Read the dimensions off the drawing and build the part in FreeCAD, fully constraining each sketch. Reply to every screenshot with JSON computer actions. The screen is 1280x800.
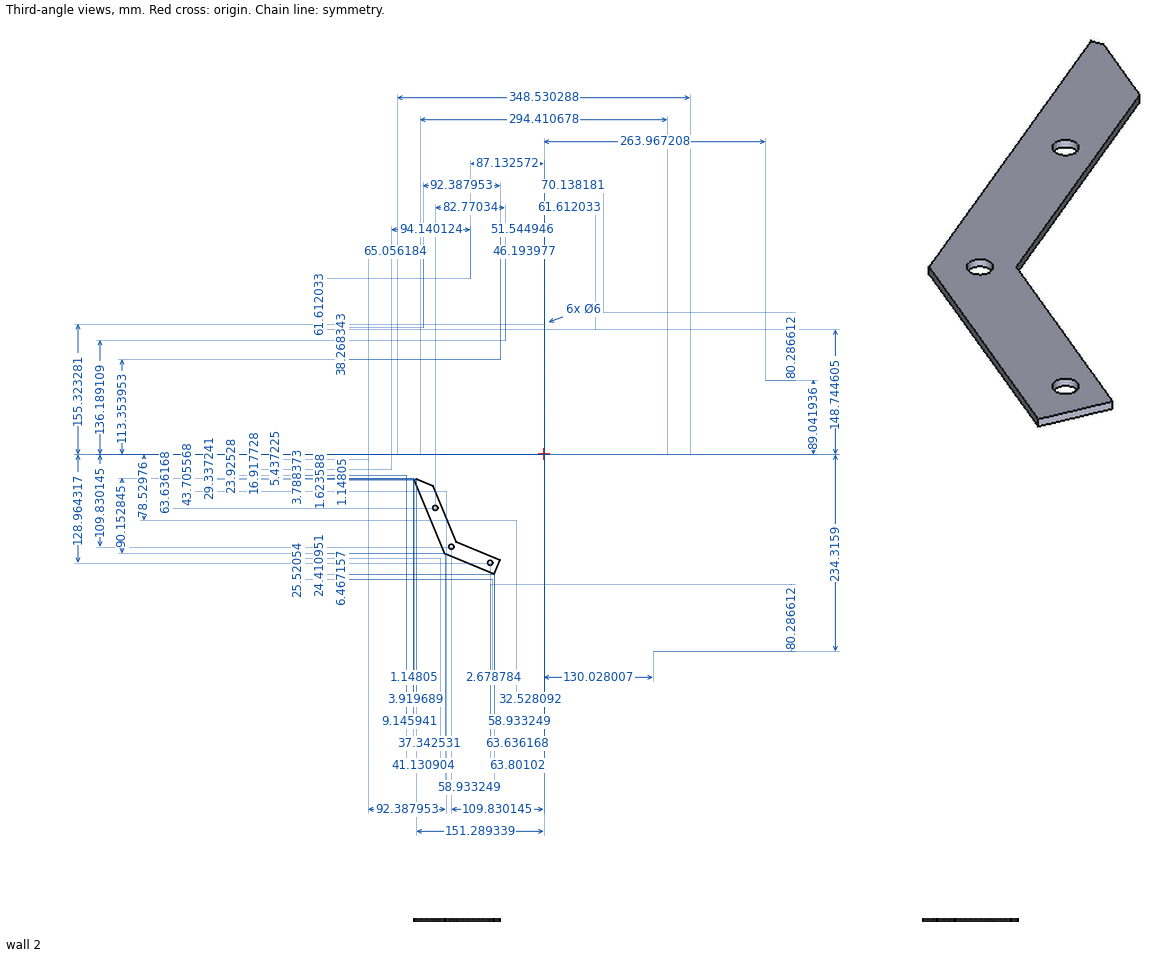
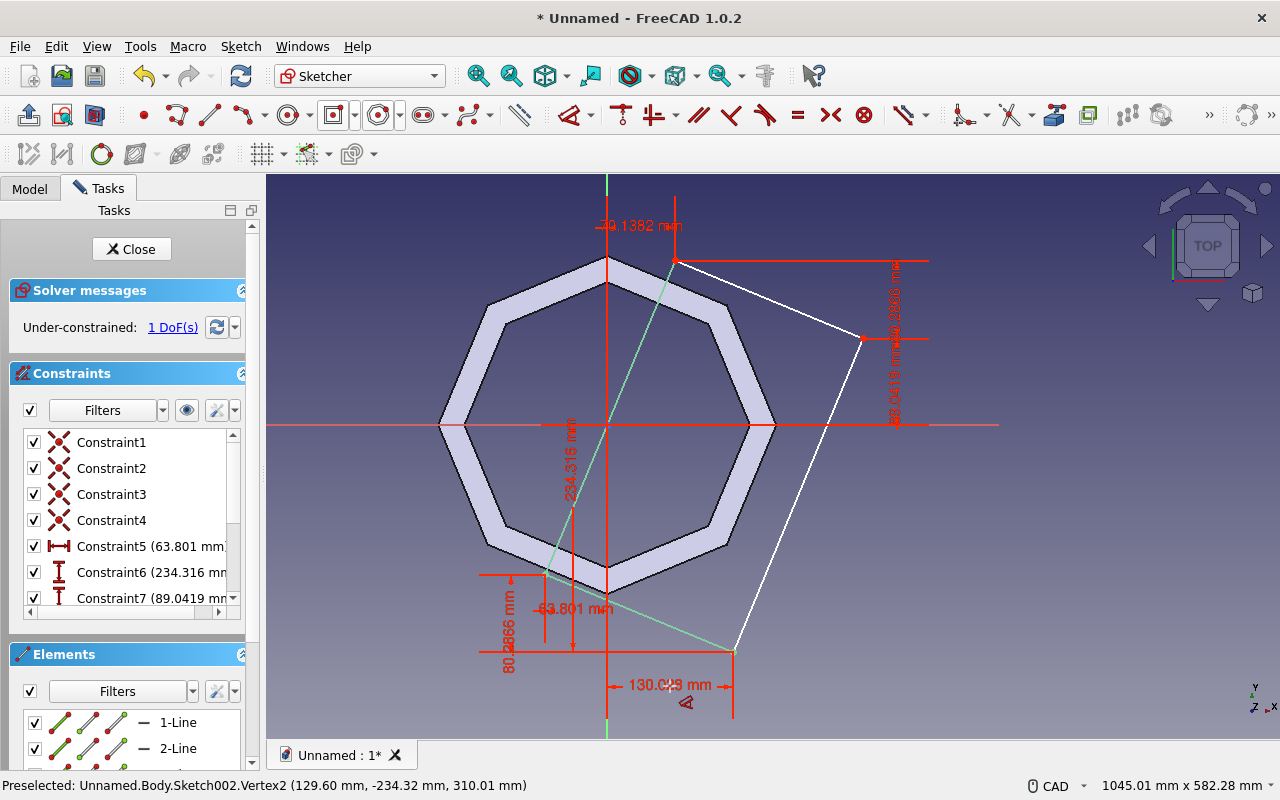
{"action": "left_click", "coordinate": [863, 339]}
{"action": "left_click", "coordinate": [735, 305]}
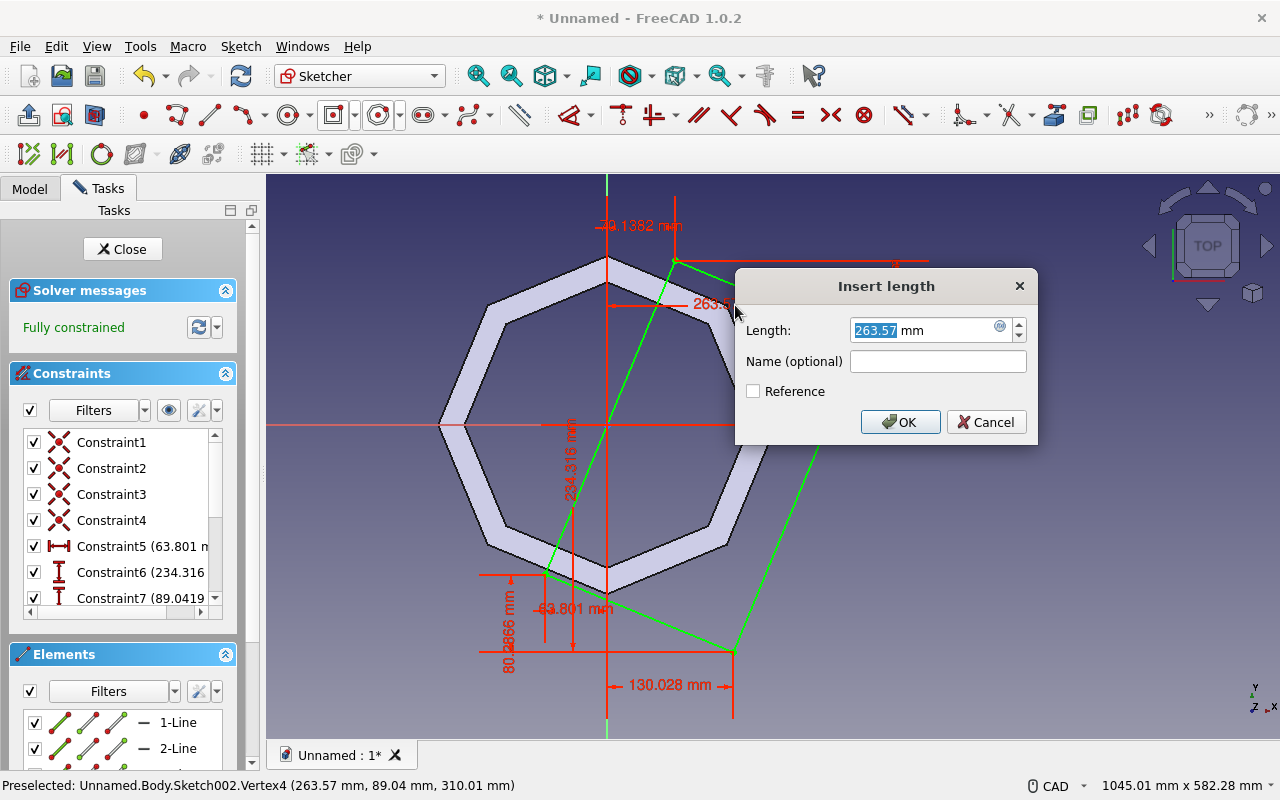
{"action": "type", "text": "263.967208"}
{"action": "key", "text": "Return"}
{"action": "key", "text": "Escape"}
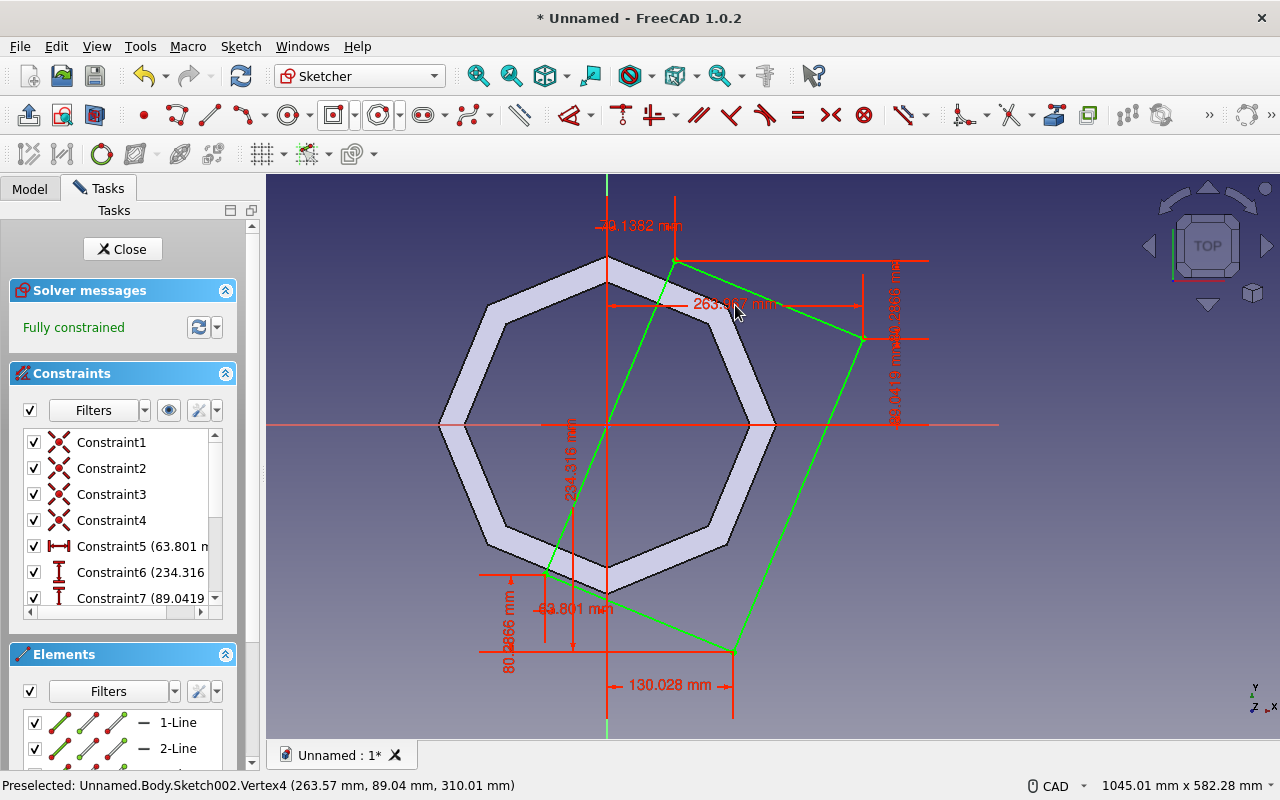
{"action": "left_click", "coordinate": [123, 249]}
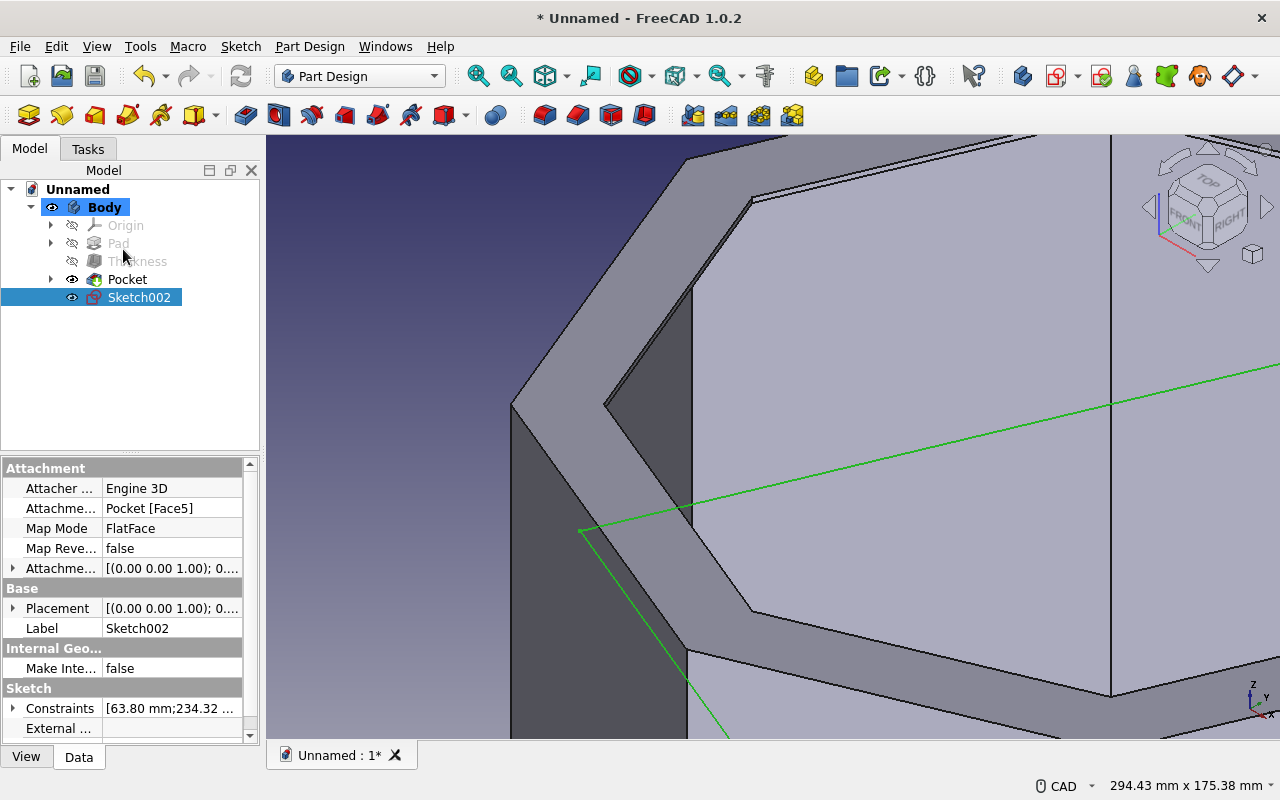
{"action": "left_click", "coordinate": [246, 116]}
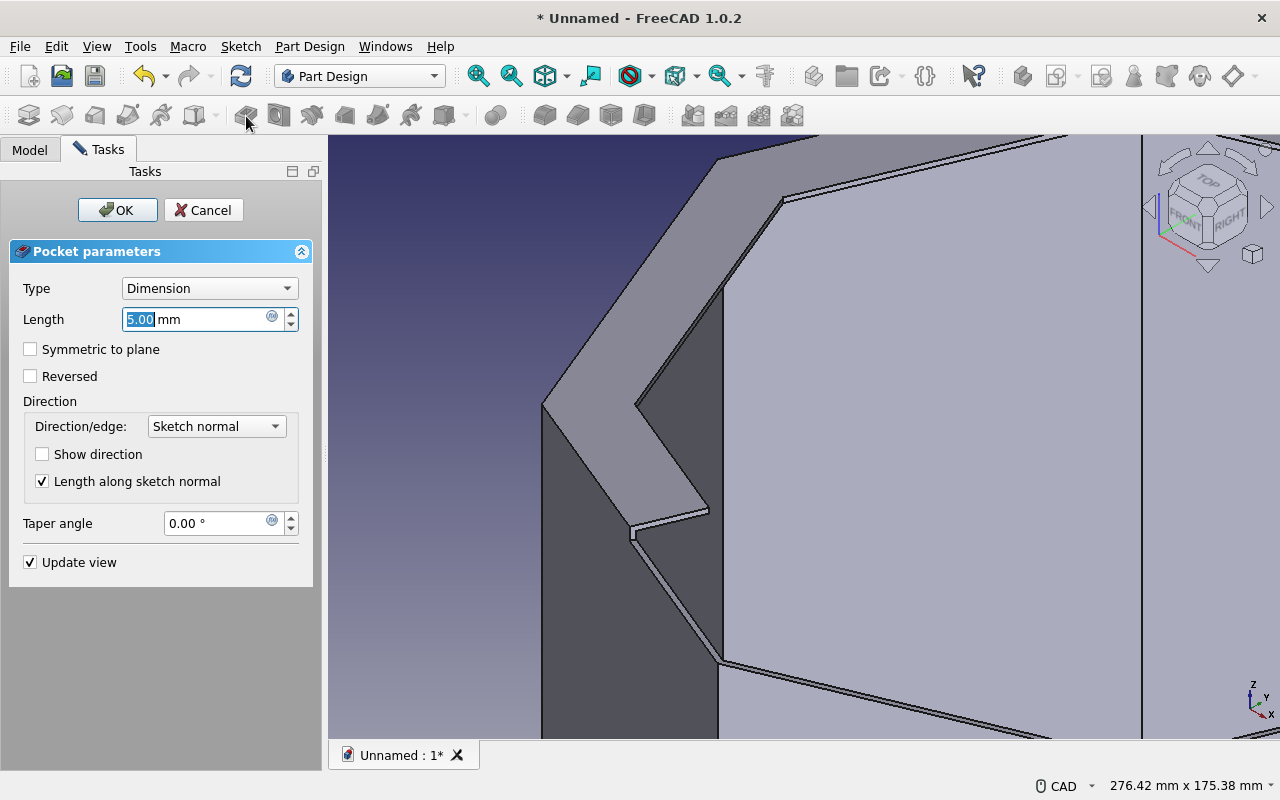
{"action": "left_click", "coordinate": [210, 288]}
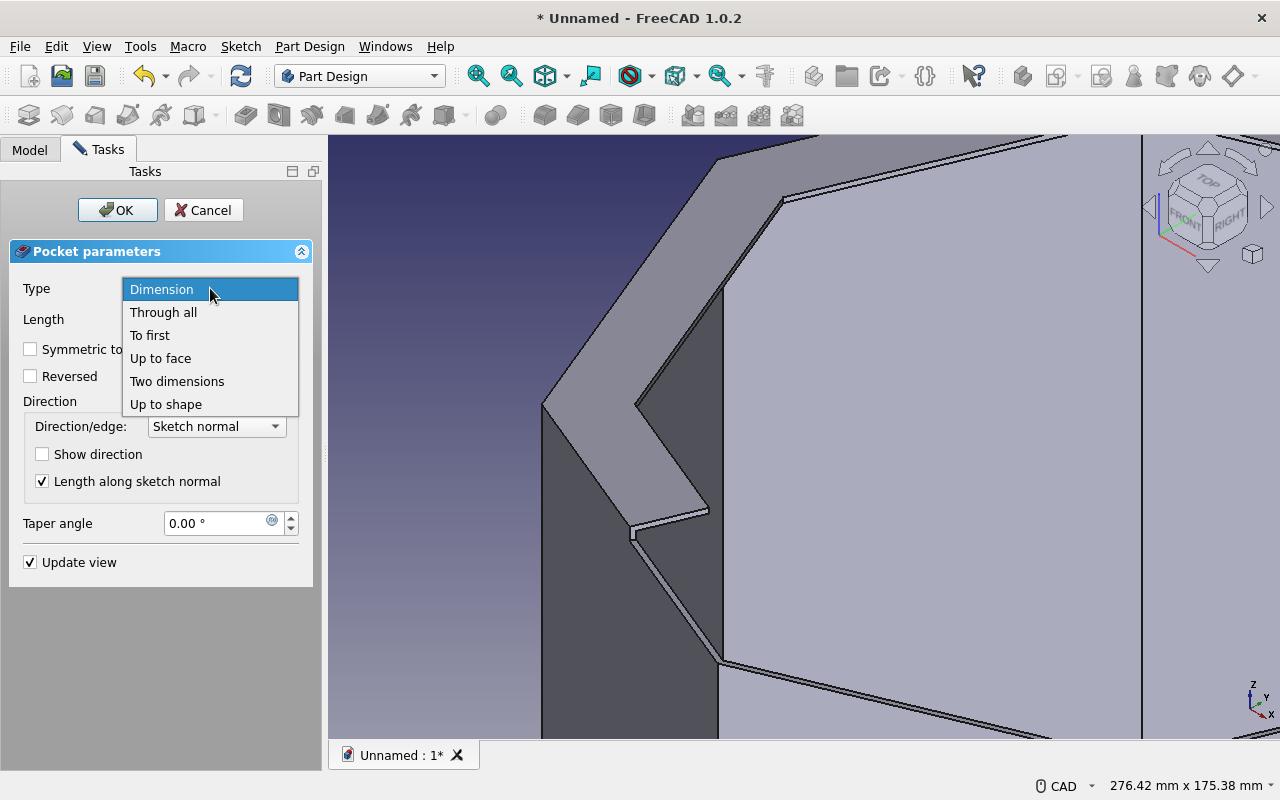
{"action": "left_click", "coordinate": [208, 312]}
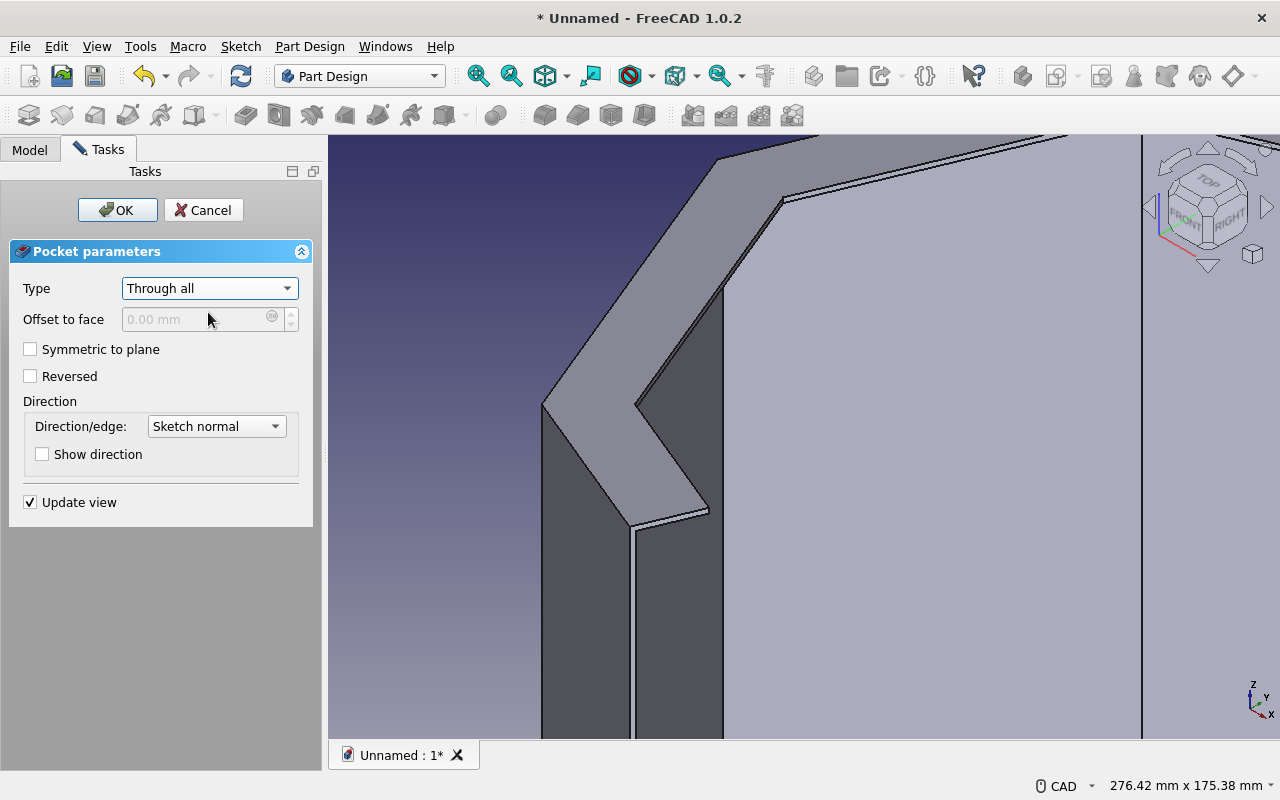
{"action": "left_click", "coordinate": [118, 210]}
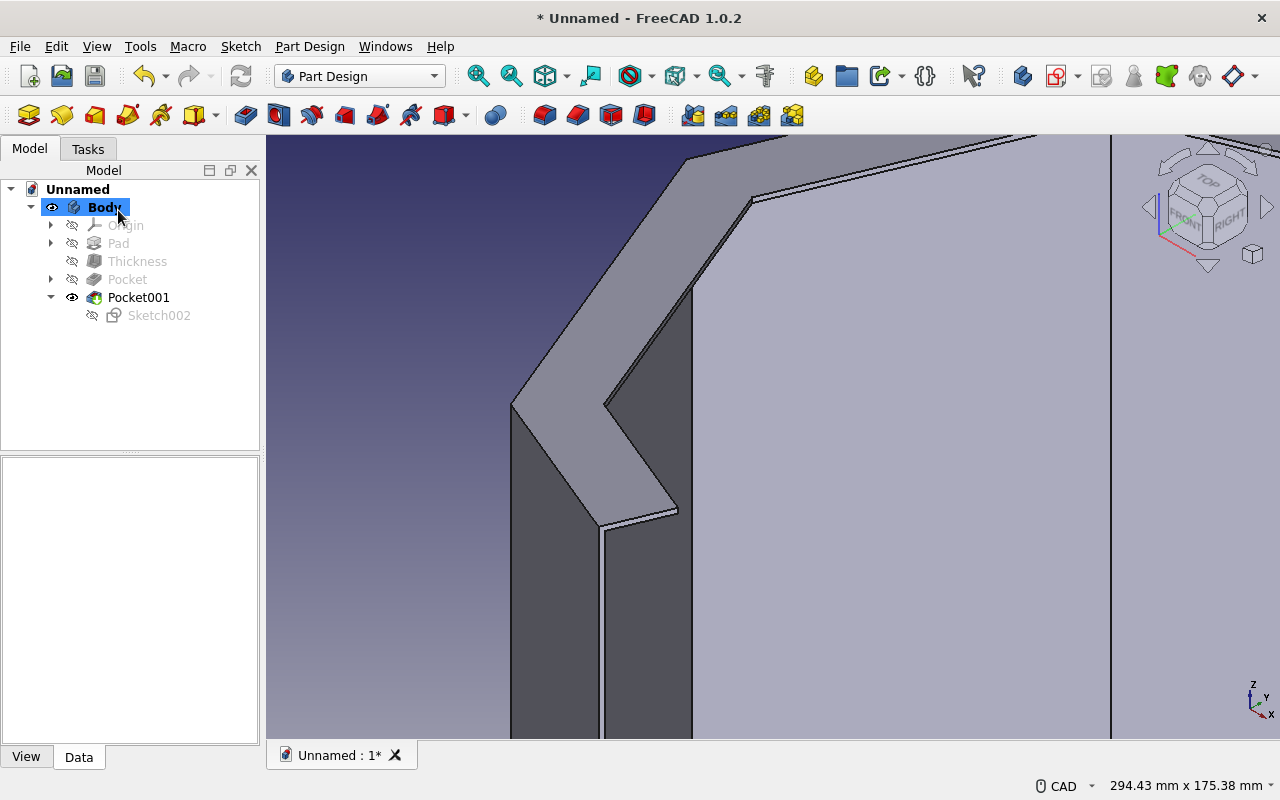
{"action": "left_click", "coordinate": [479, 76]}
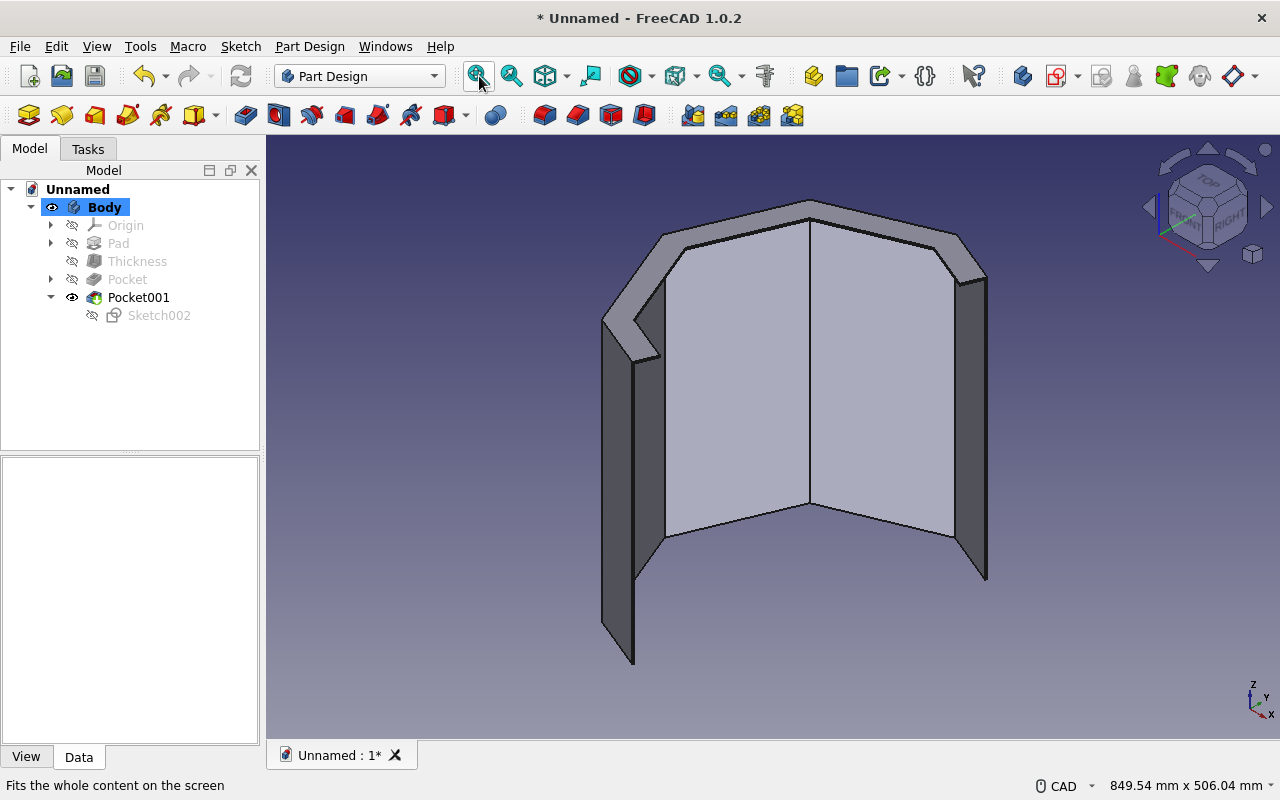
{"action": "left_click", "coordinate": [918, 234]}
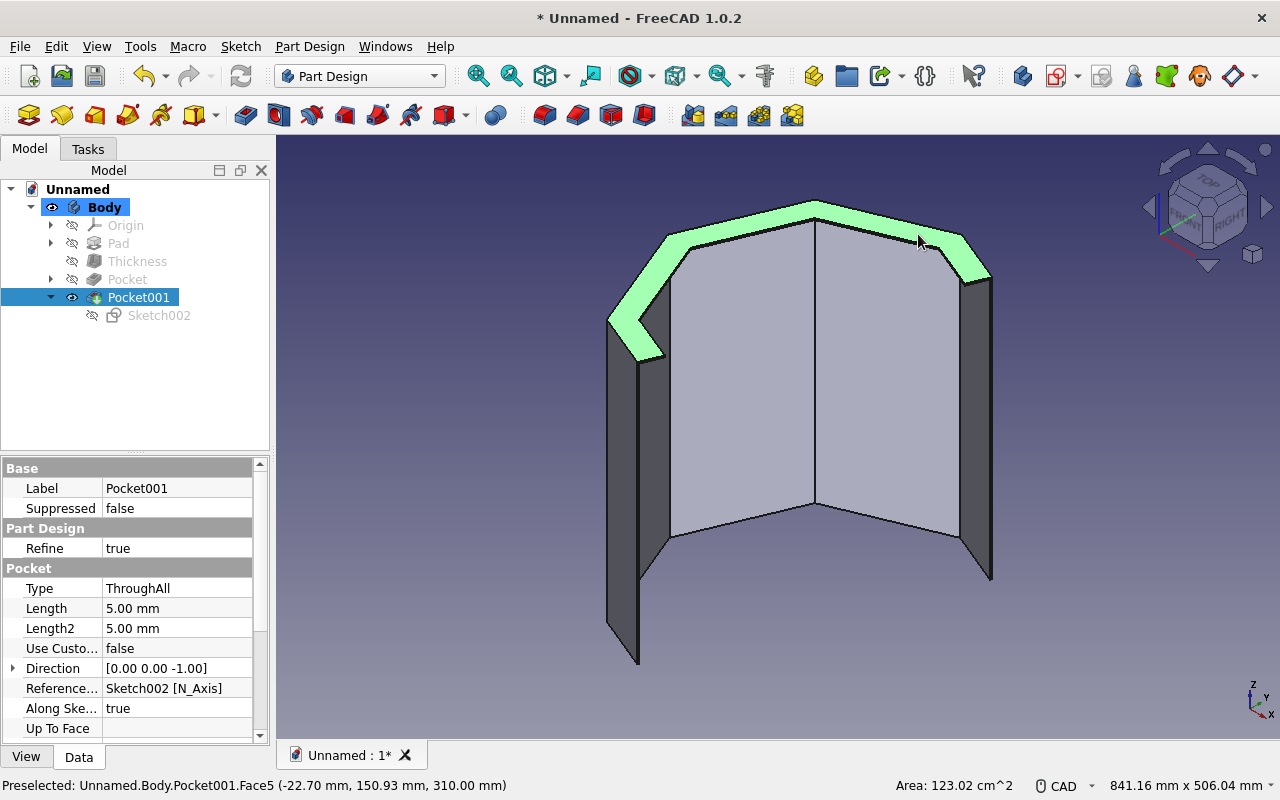
{"action": "left_click", "coordinate": [1056, 76]}